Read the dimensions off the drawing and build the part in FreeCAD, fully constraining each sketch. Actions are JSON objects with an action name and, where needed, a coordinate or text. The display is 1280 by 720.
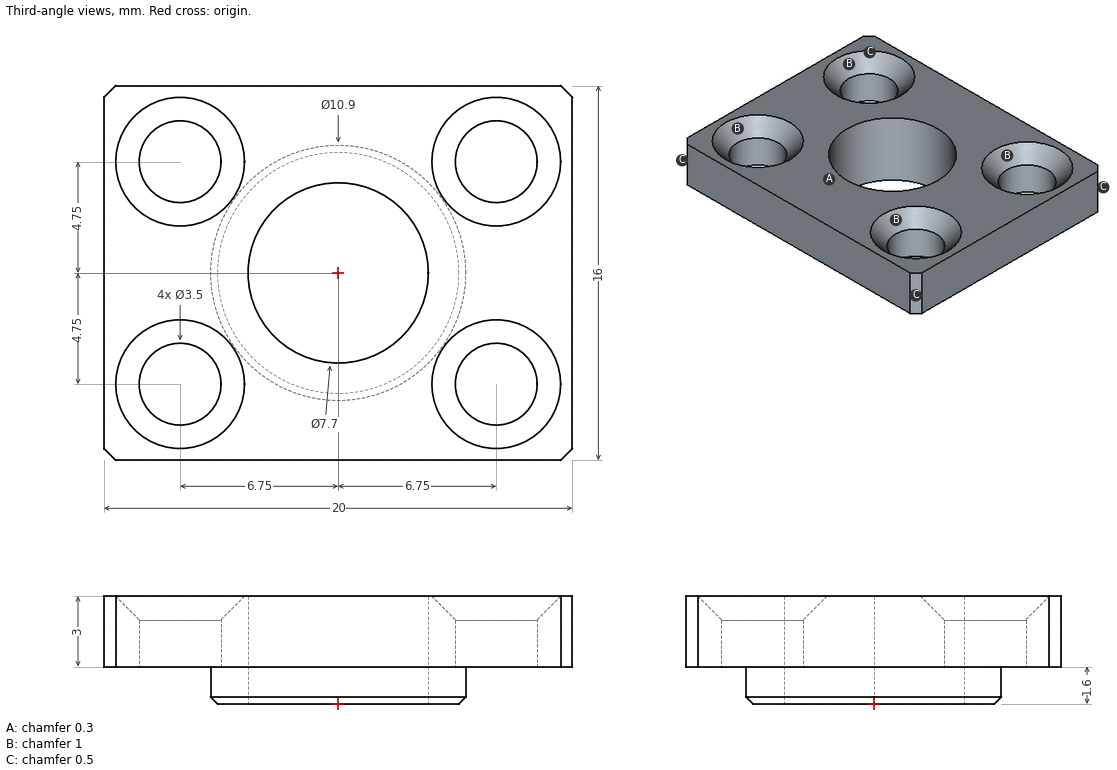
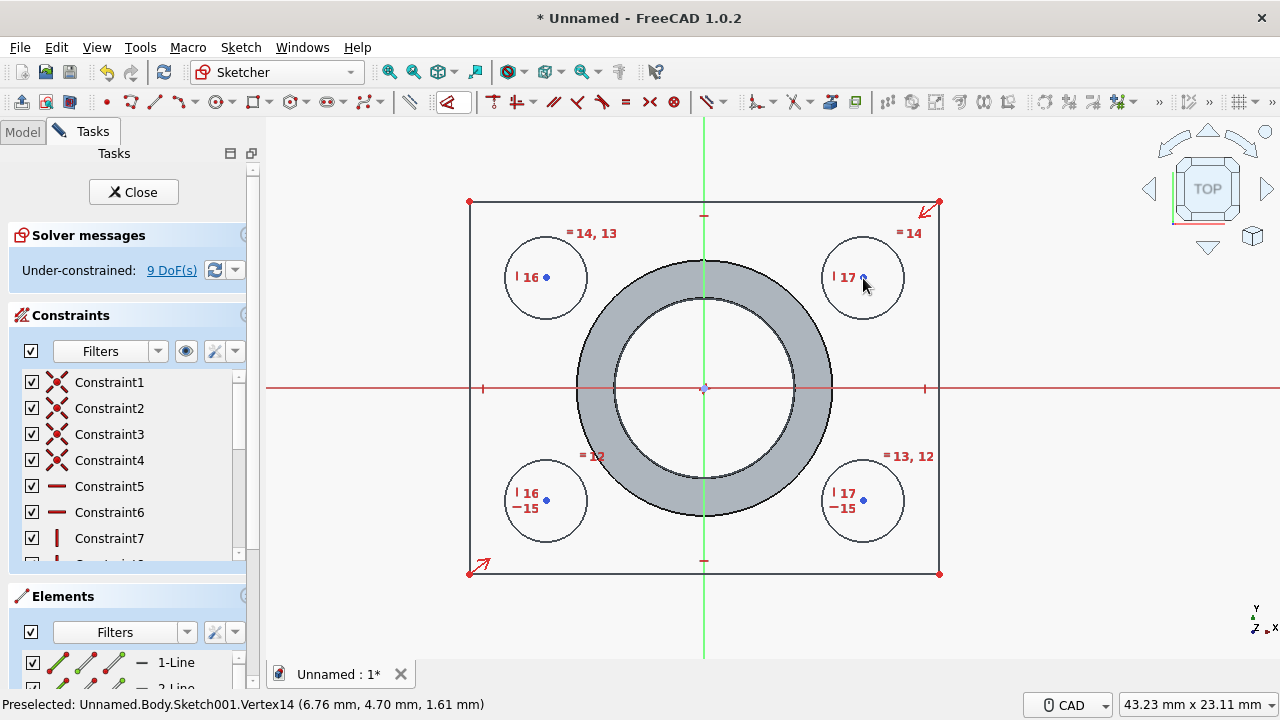
{"action": "left_click", "coordinate": [575, 472]}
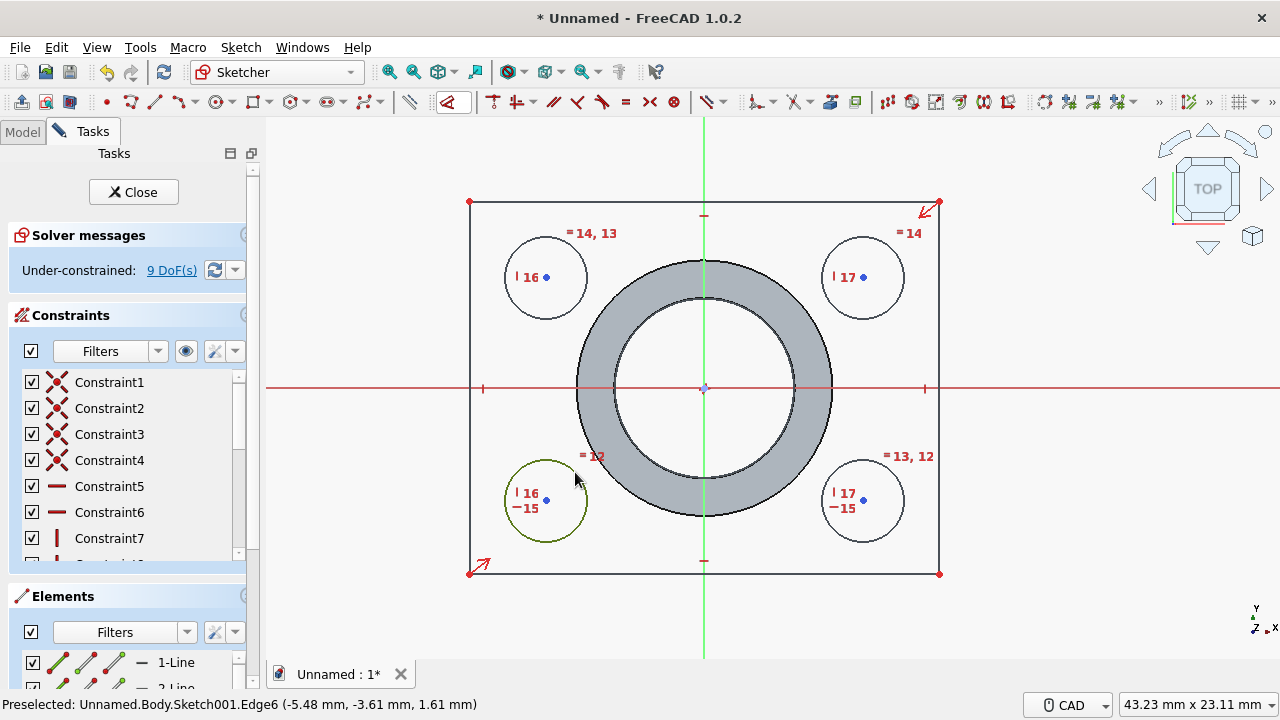
{"action": "key", "text": "k o"}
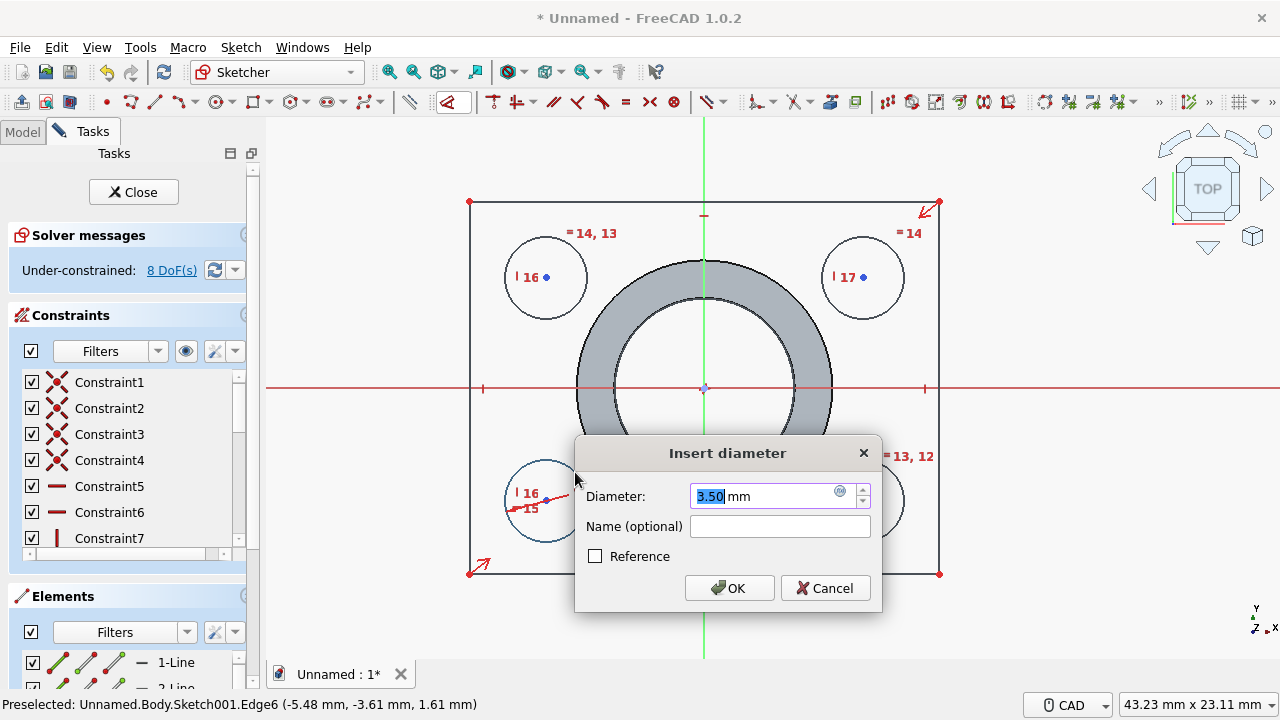
{"action": "type", "text": "3.5"}
{"action": "key", "text": "Return"}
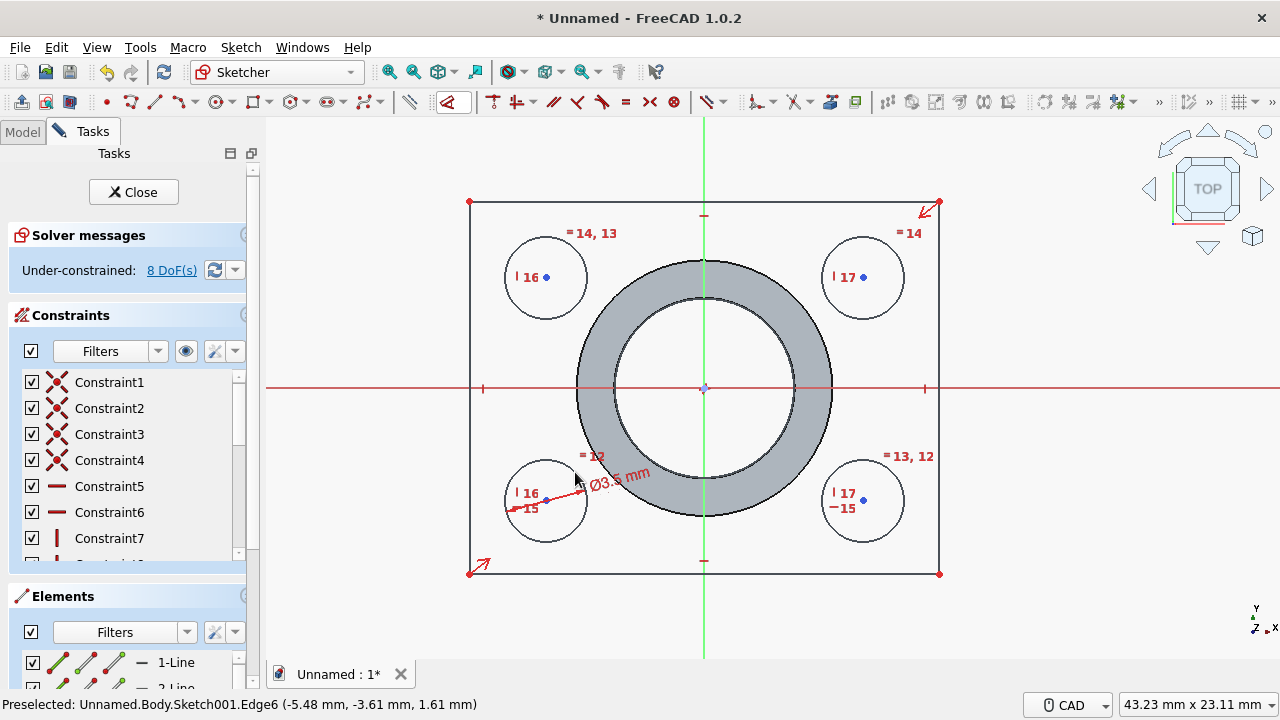
{"action": "left_click", "coordinate": [768, 325]}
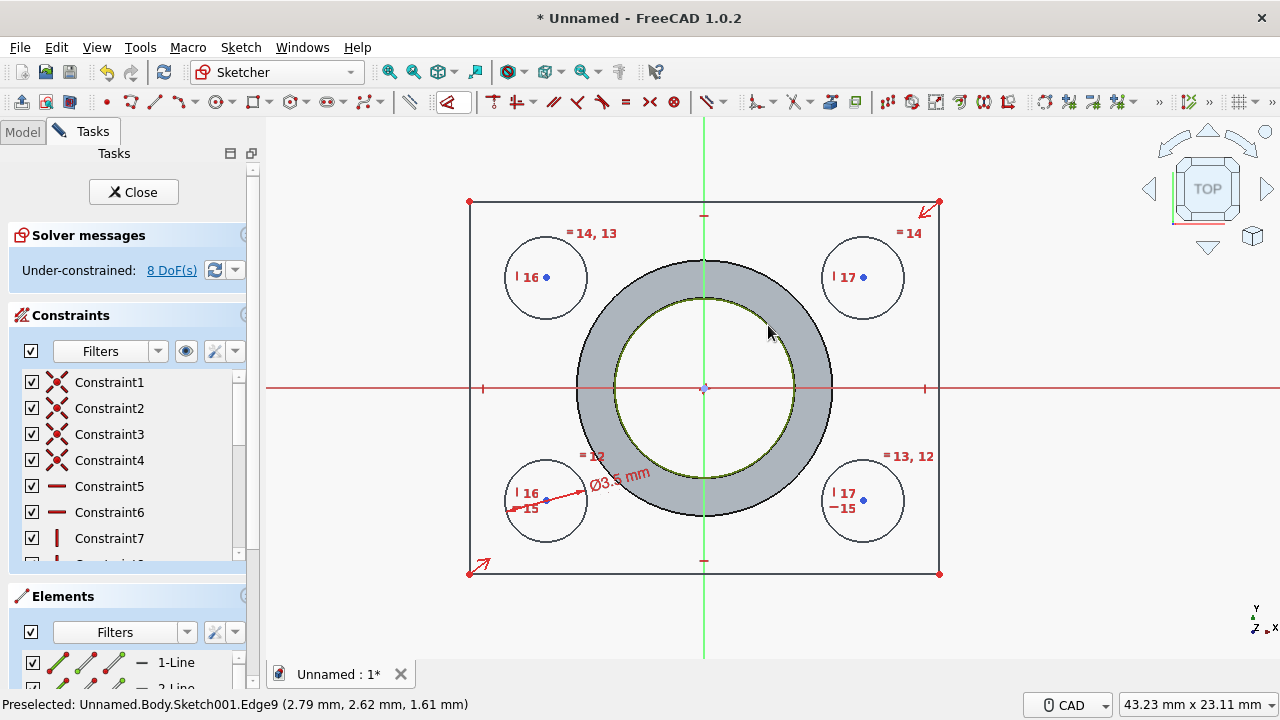
{"action": "key", "text": "k o"}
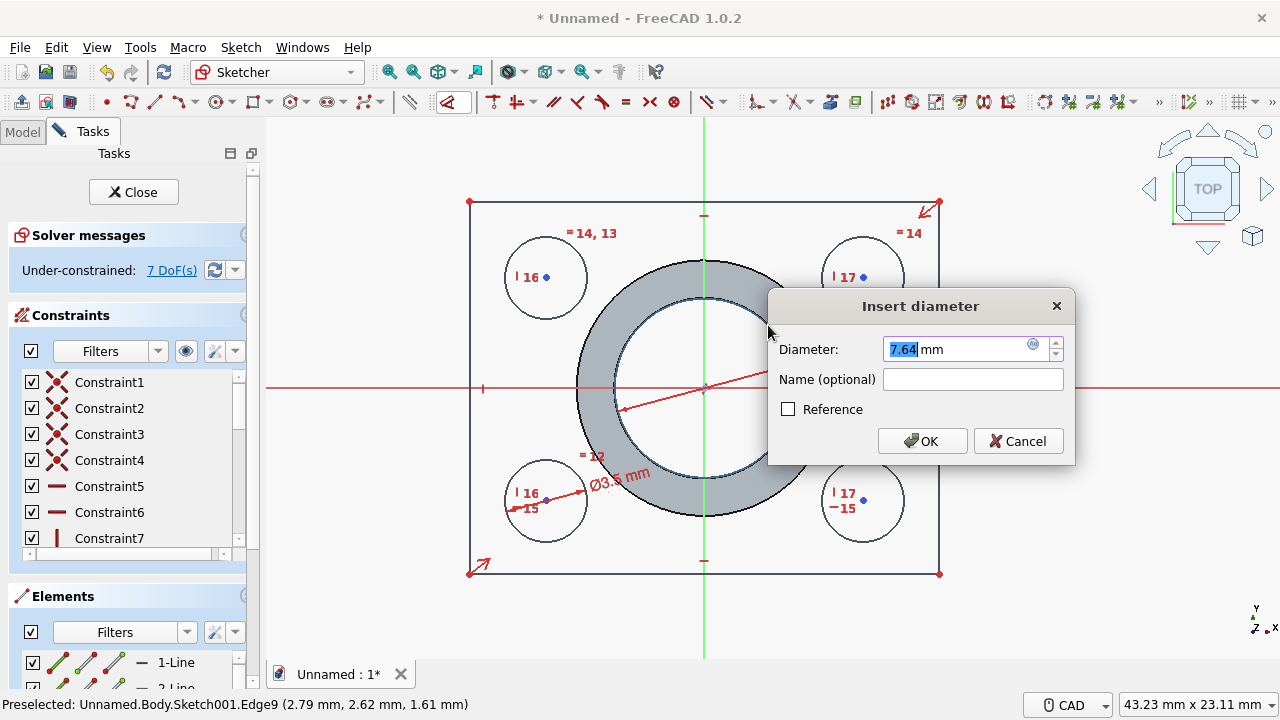
{"action": "type", "text": "7.7"}
{"action": "key", "text": "Return"}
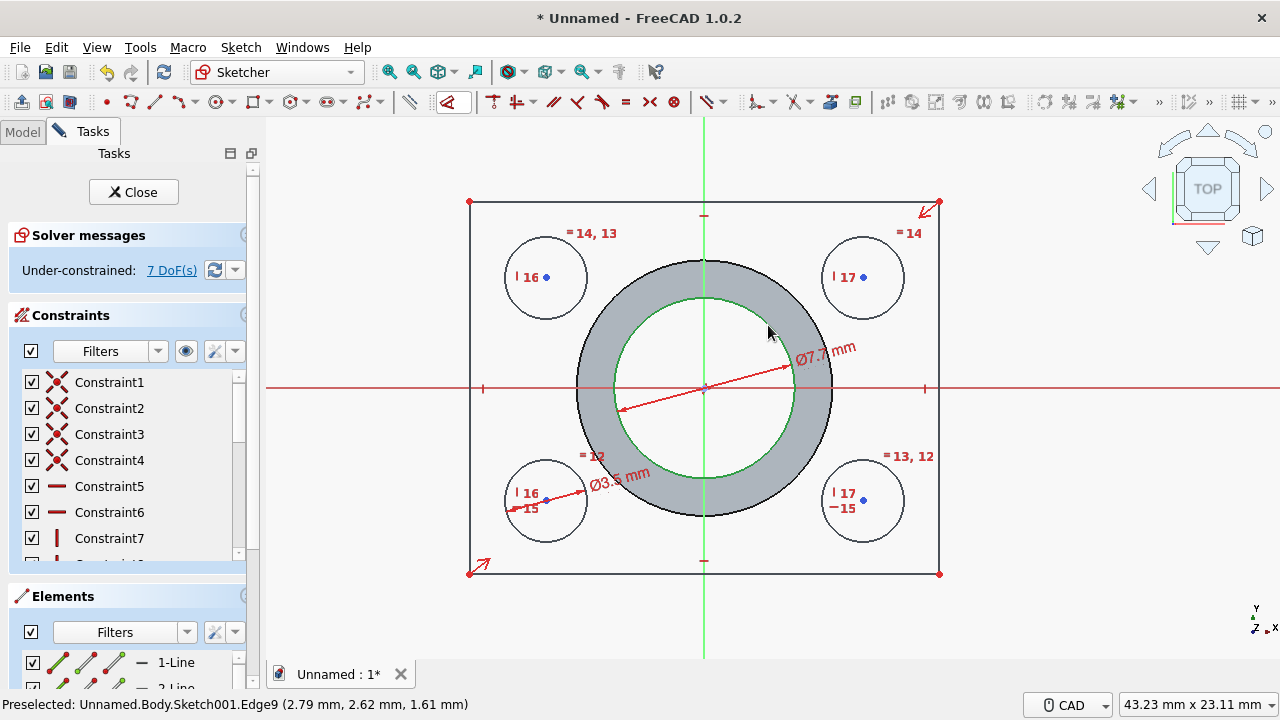
{"action": "left_click", "coordinate": [611, 574]}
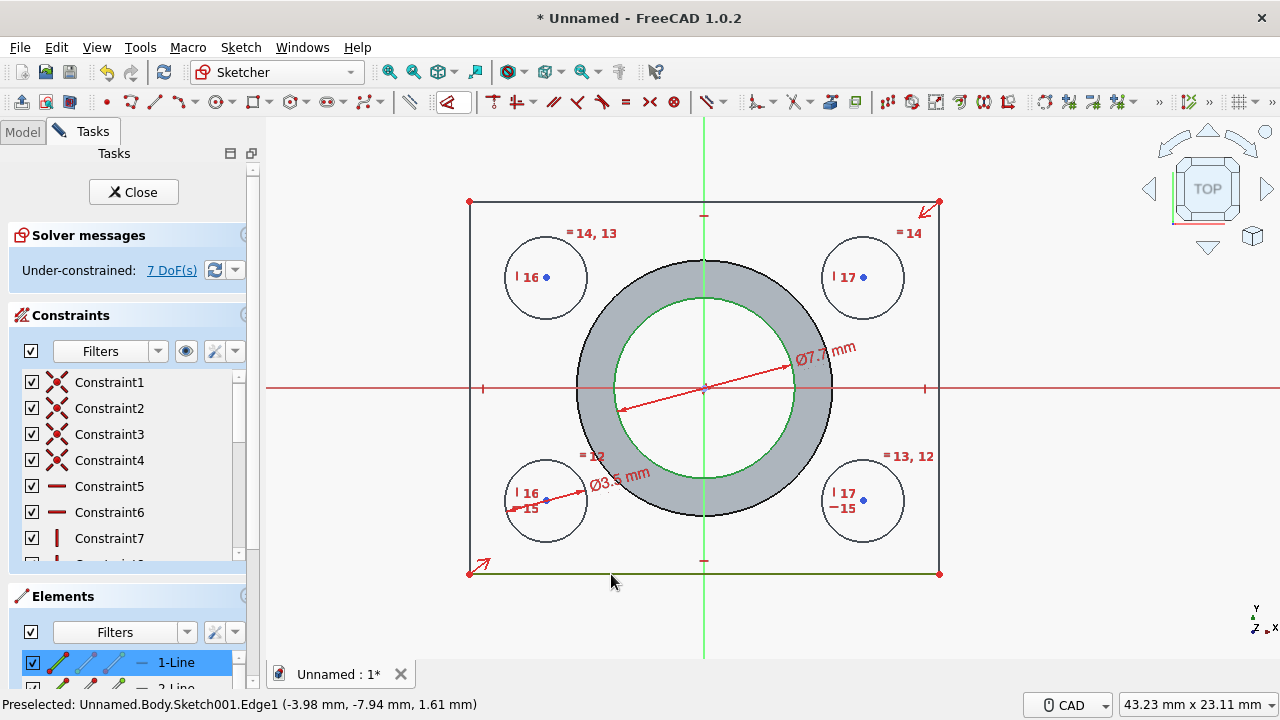
{"action": "key", "text": "l"}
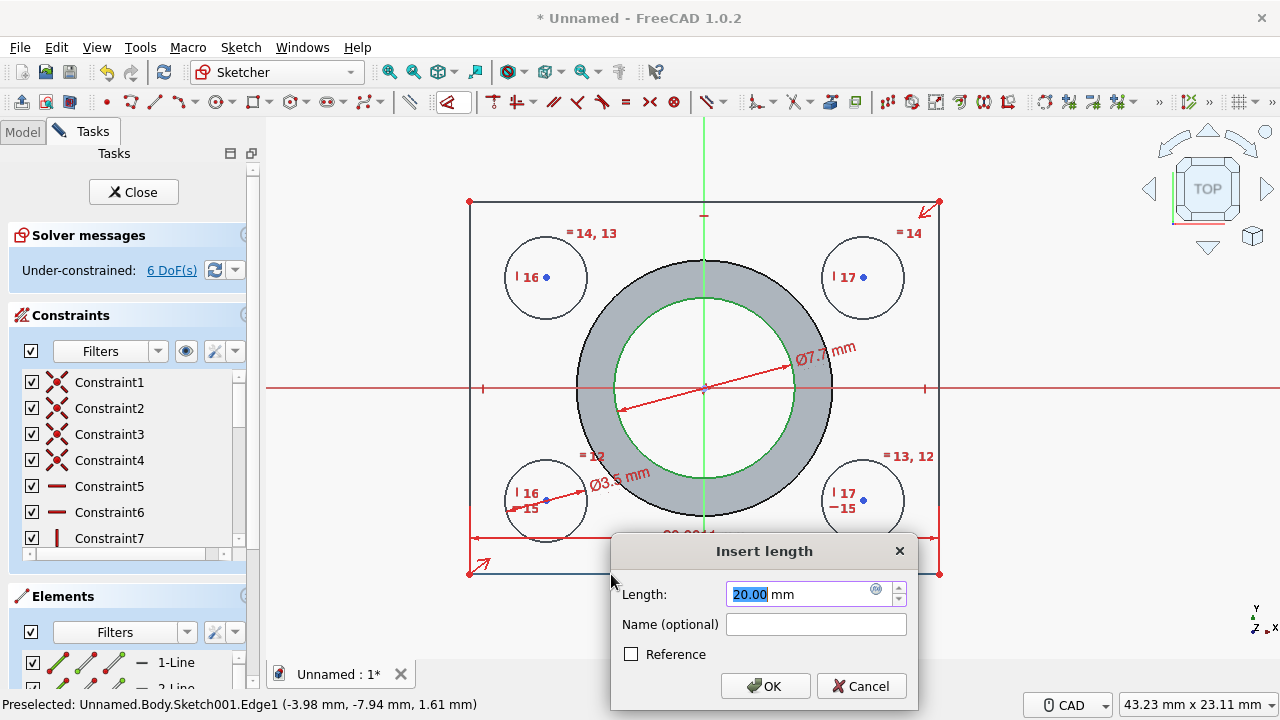
{"action": "type", "text": "20"}
{"action": "key", "text": "Return"}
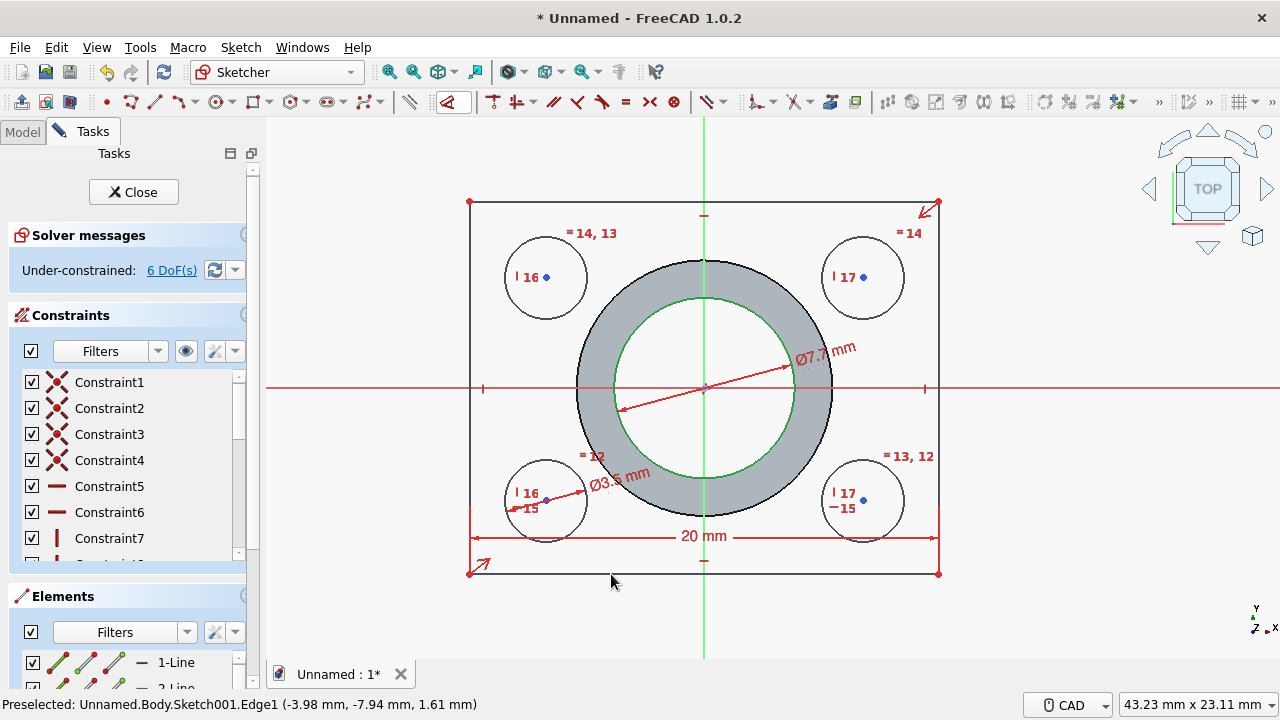
{"action": "left_click", "coordinate": [939, 463]}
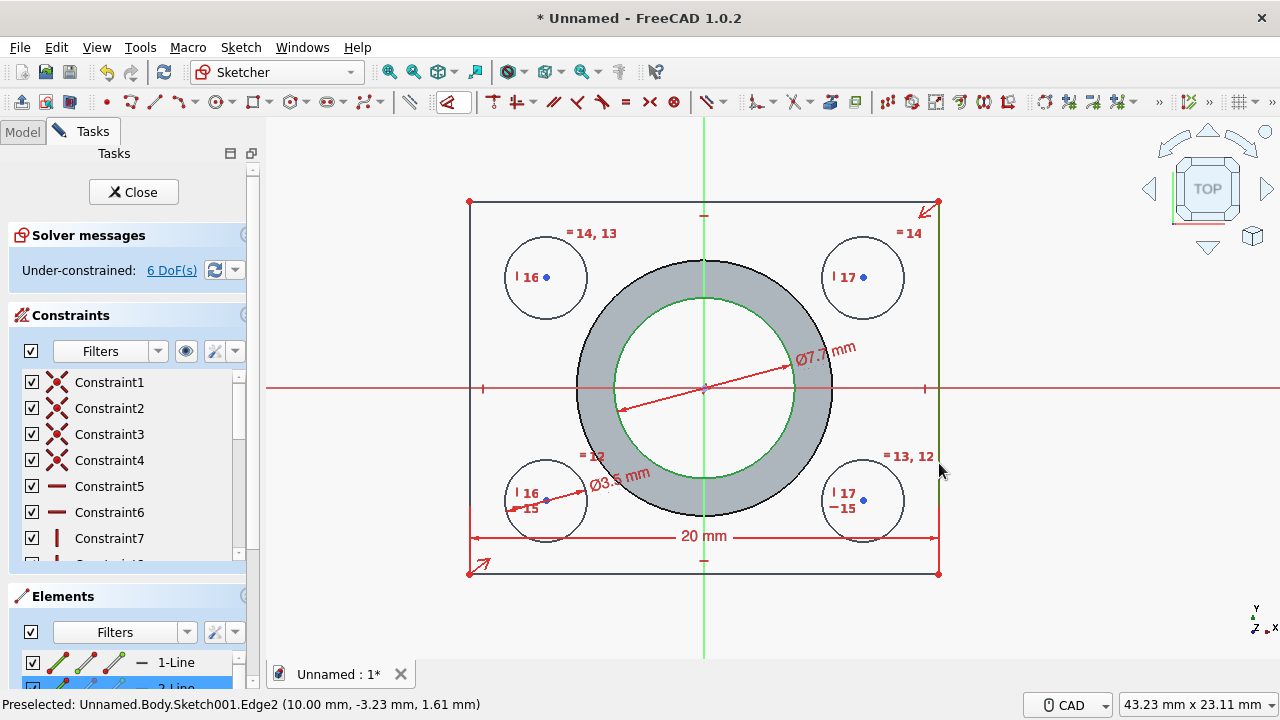
{"action": "key", "text": "i"}